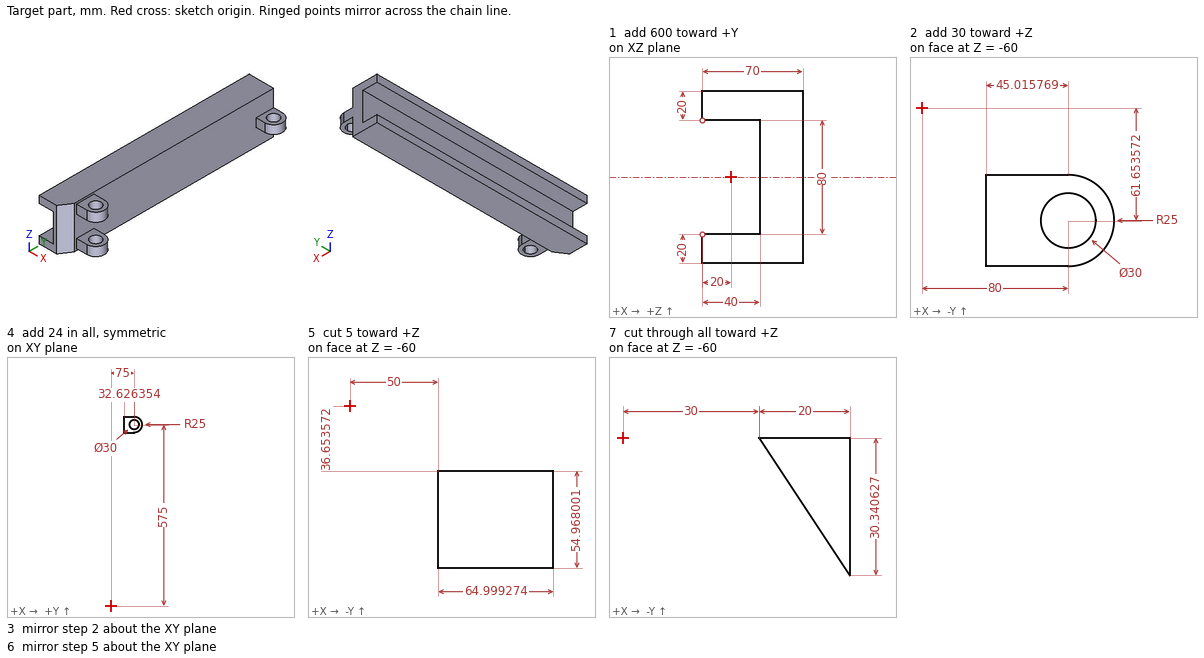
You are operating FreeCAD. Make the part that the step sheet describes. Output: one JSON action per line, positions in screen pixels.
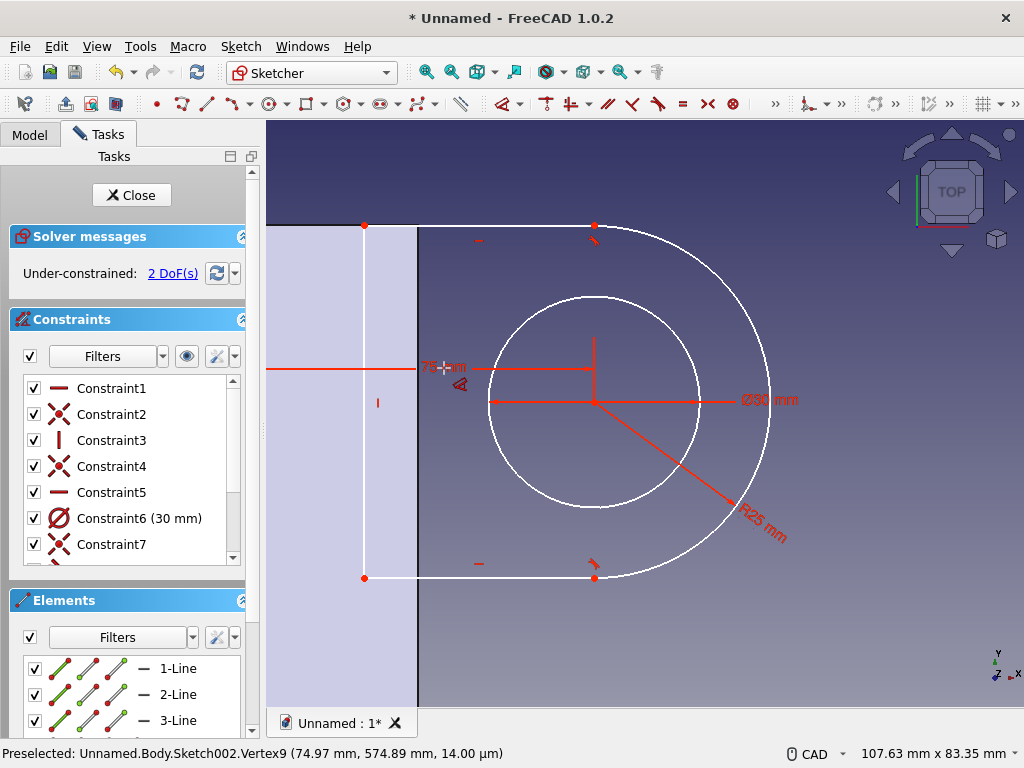
{"action": "left_click", "coordinate": [594, 402]}
{"action": "left_click", "coordinate": [628, 541]}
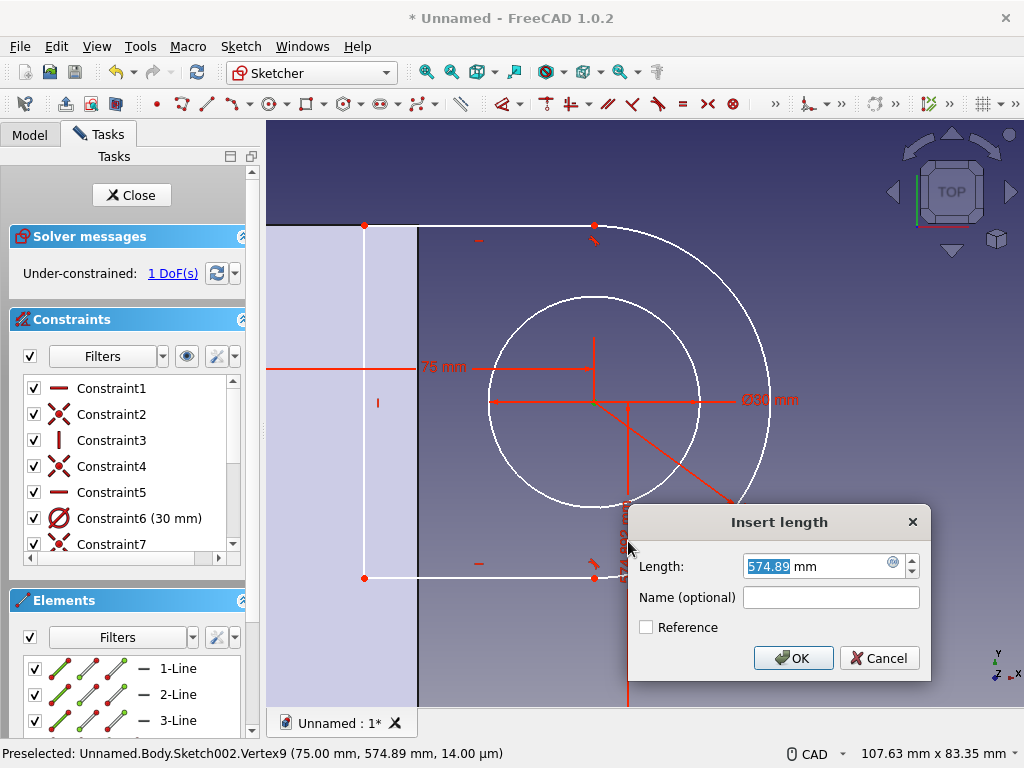
{"action": "type", "text": "575"}
{"action": "key", "text": "Return"}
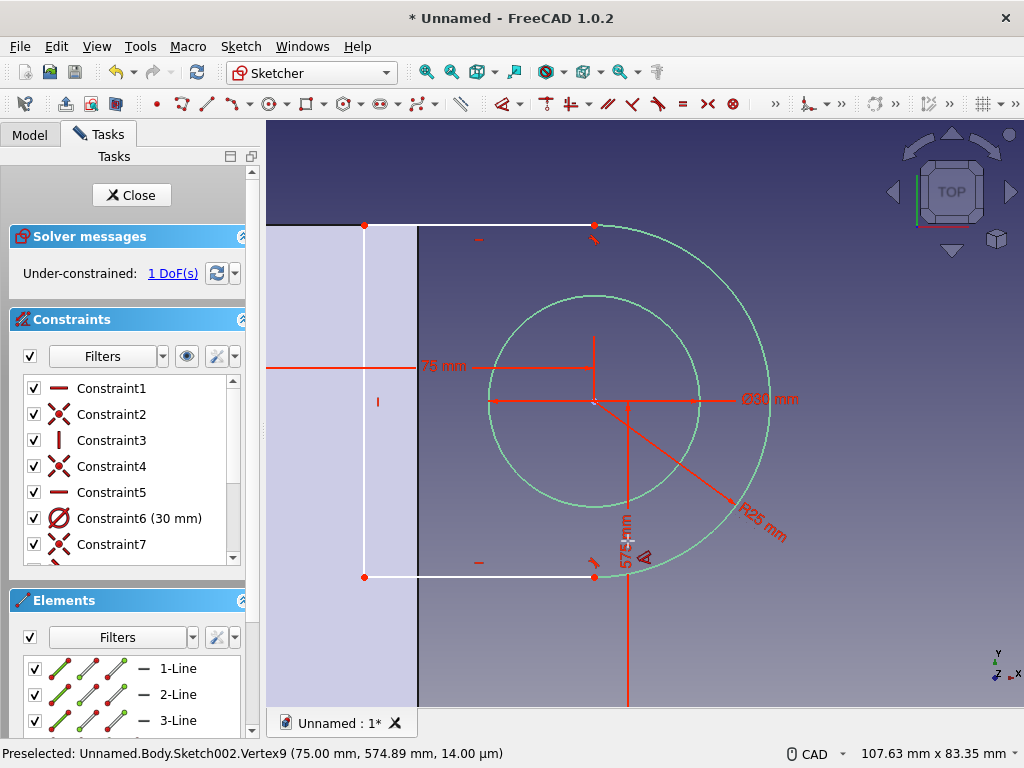
{"action": "left_click", "coordinate": [525, 225]}
{"action": "left_click", "coordinate": [479, 191]}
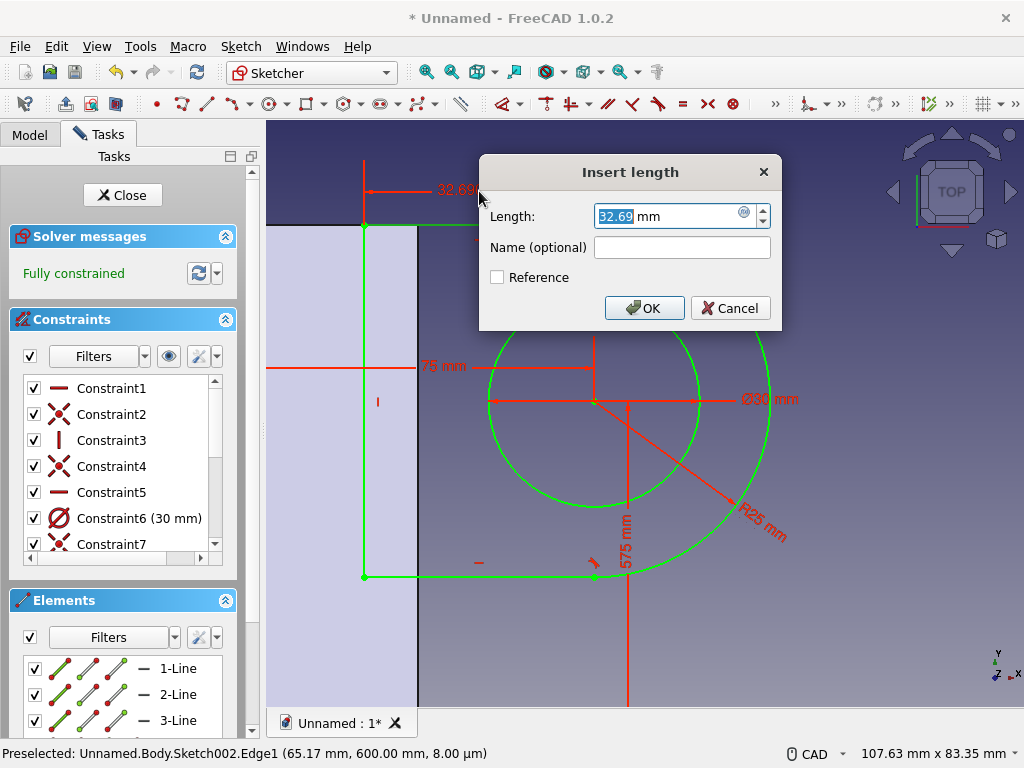
{"action": "type", "text": "32.626354"}
{"action": "key", "text": "Return"}
{"action": "key", "text": "Escape"}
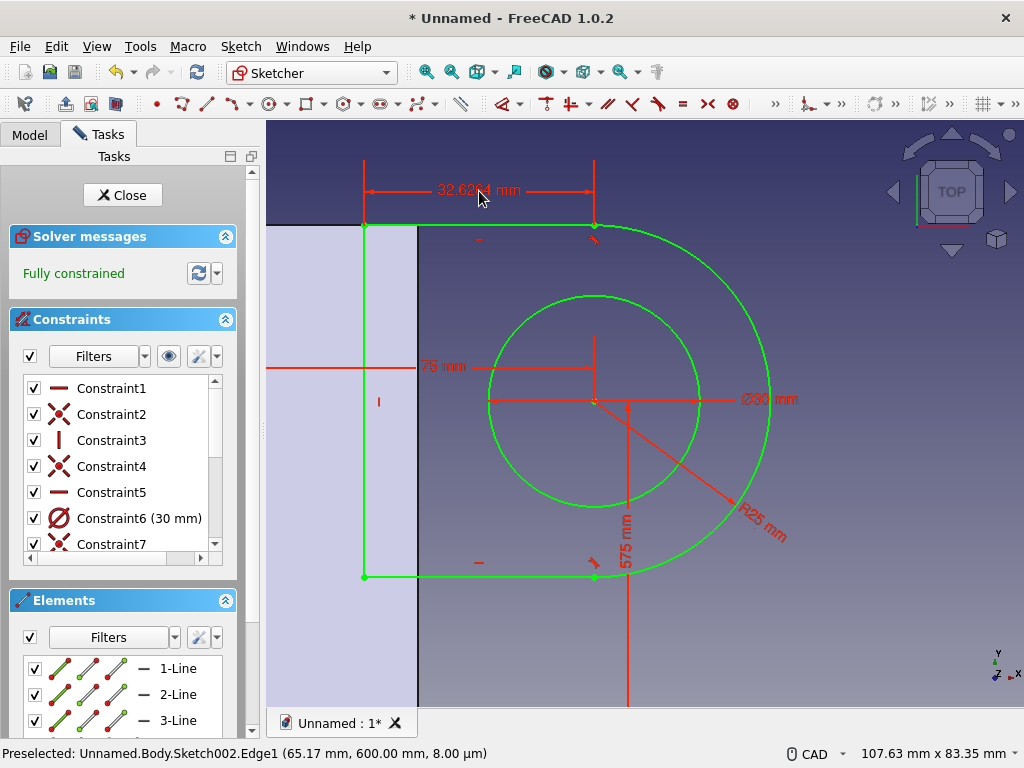
{"action": "left_click", "coordinate": [123, 195]}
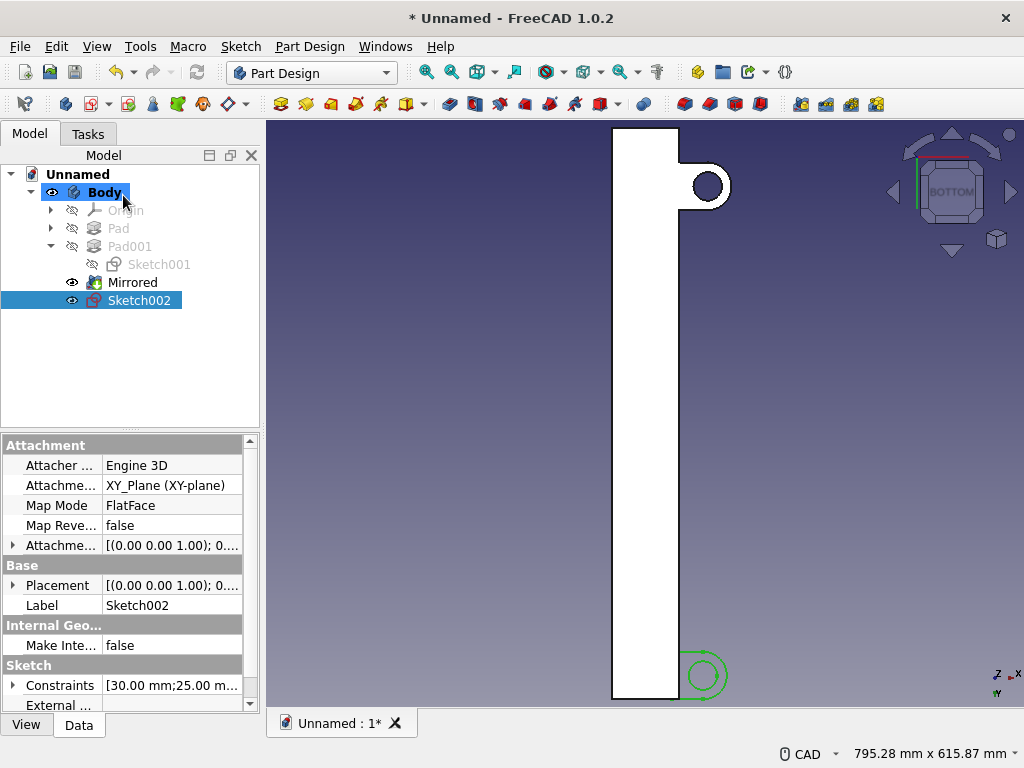
{"action": "left_click", "coordinate": [281, 104]}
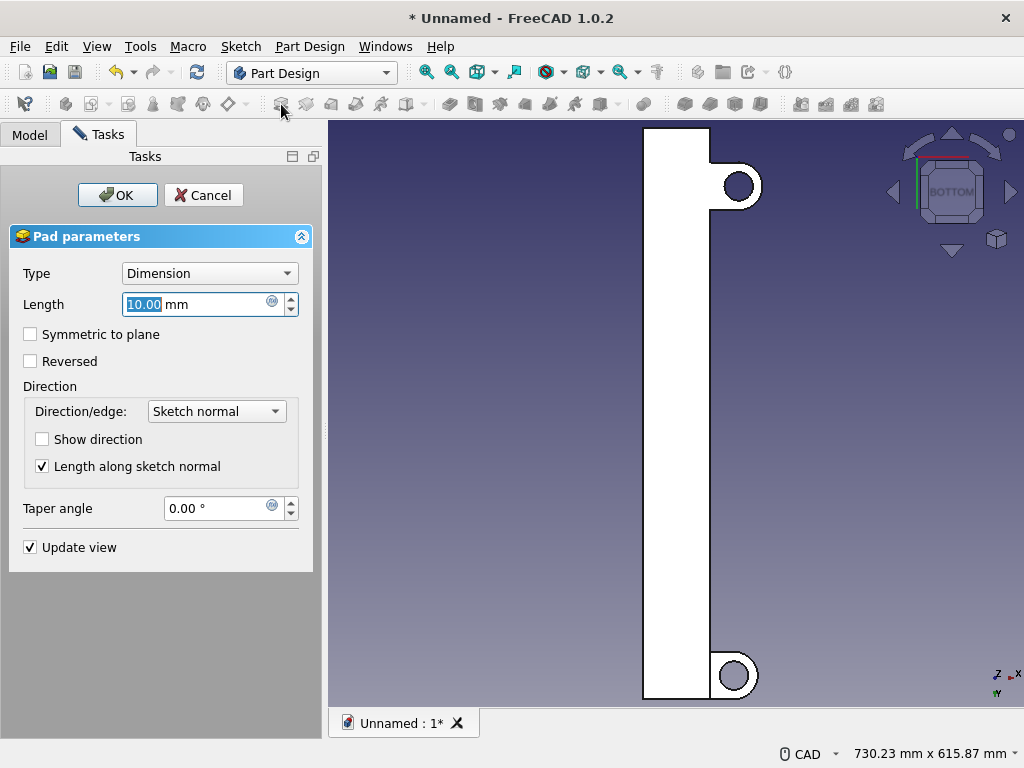
{"action": "type", "text": "24"}
{"action": "key", "text": "Tab"}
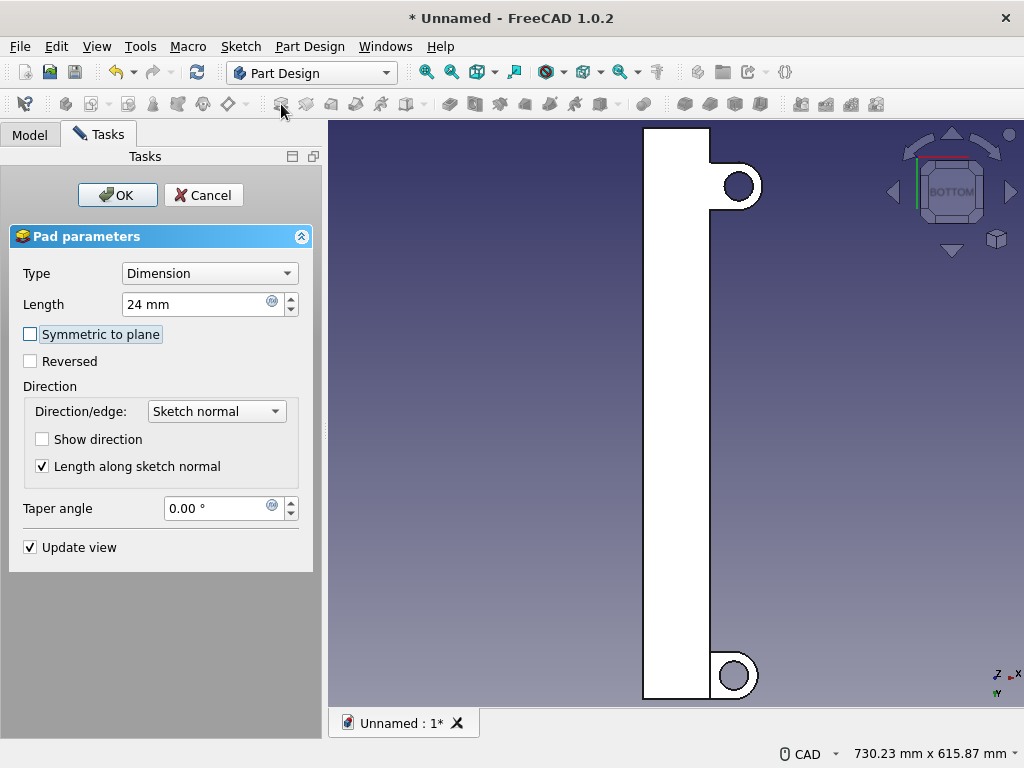
{"action": "left_click", "coordinate": [31, 334]}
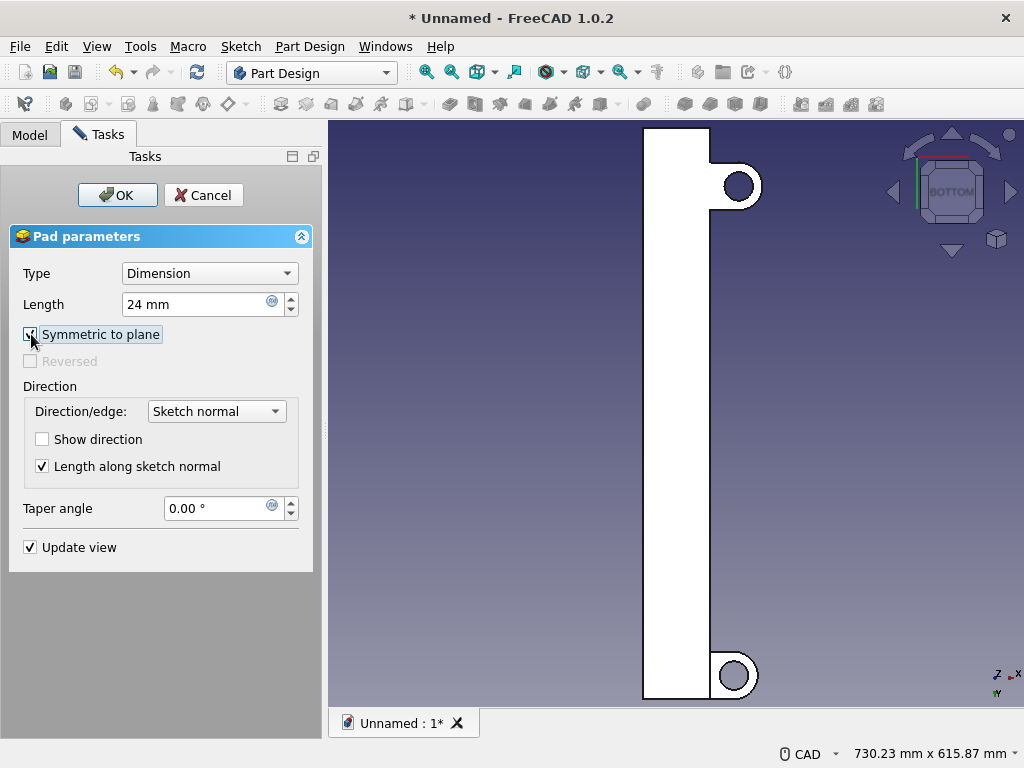
{"action": "left_click", "coordinate": [118, 195]}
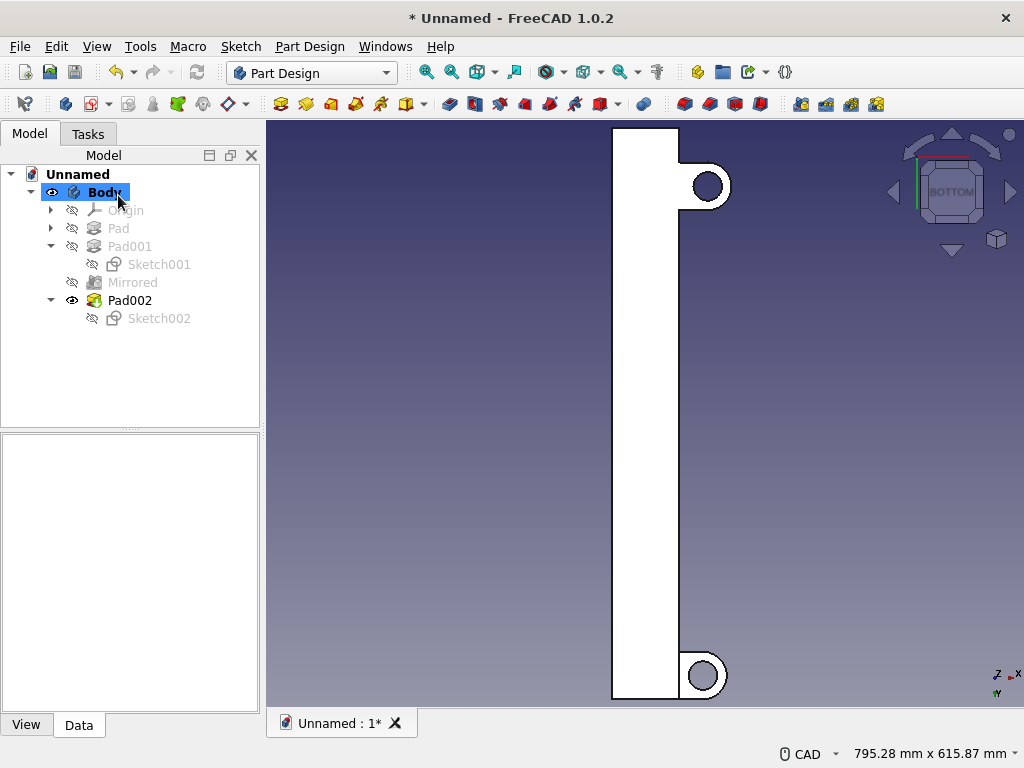
{"action": "left_click", "coordinate": [638, 658]}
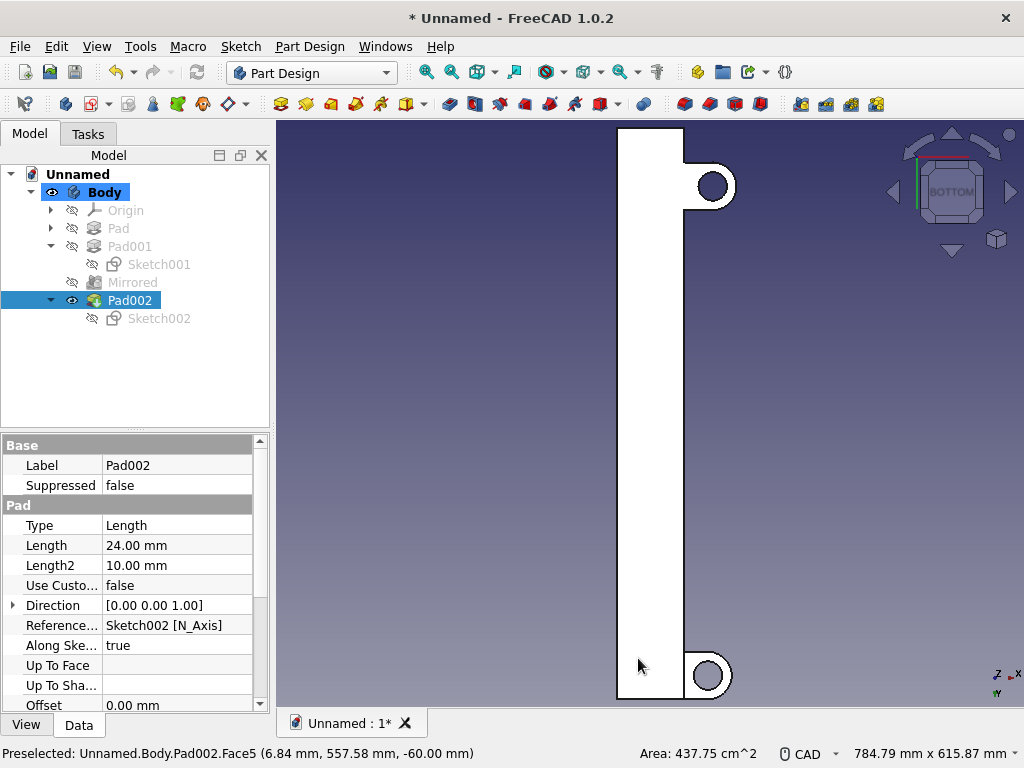
{"action": "left_click", "coordinate": [90, 104]}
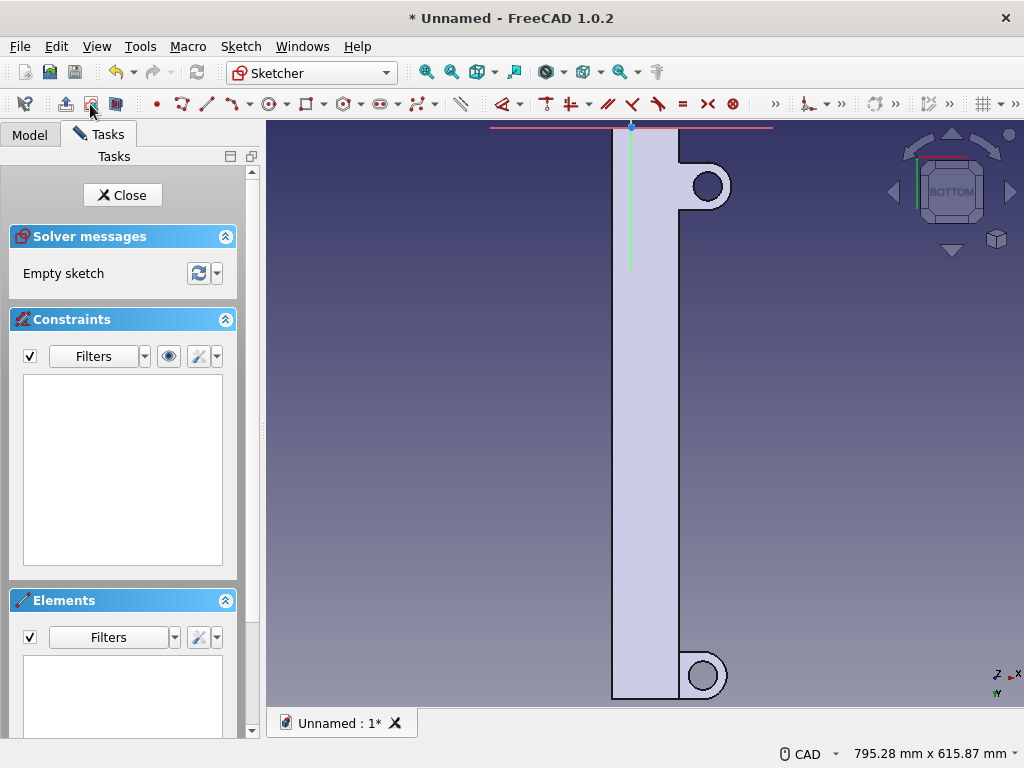
{"action": "scroll", "coordinate": [576, 414], "scroll_direction": "down", "scroll_amount": 5}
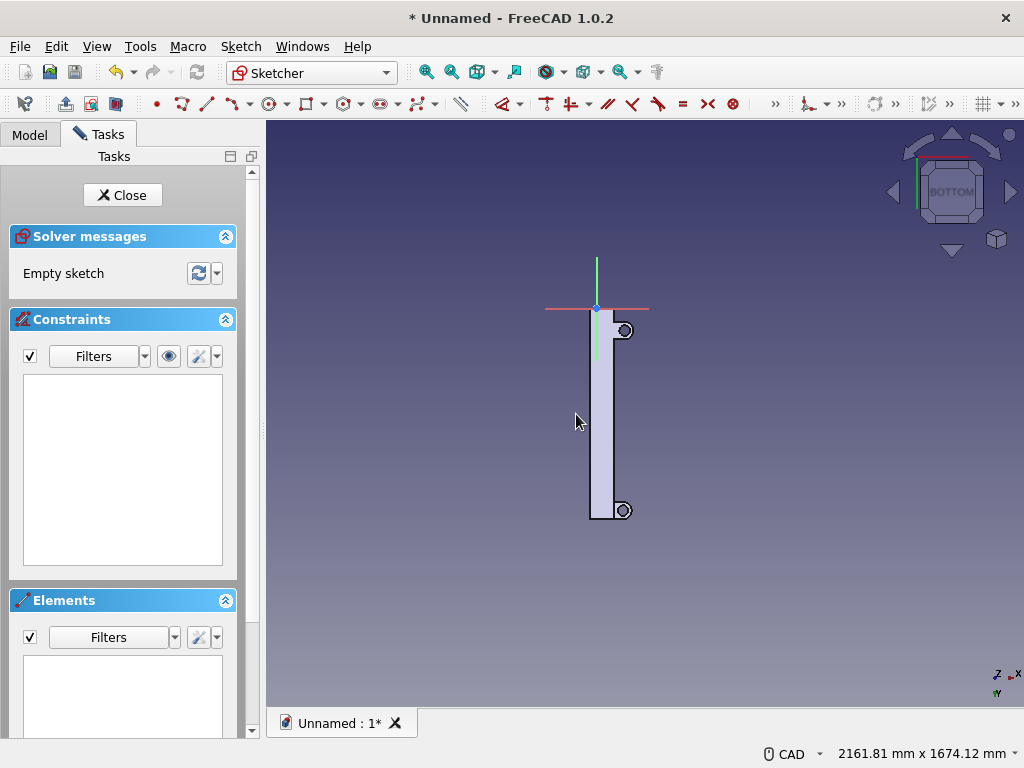
{"action": "scroll", "coordinate": [622, 314], "scroll_direction": "up", "scroll_amount": 11}